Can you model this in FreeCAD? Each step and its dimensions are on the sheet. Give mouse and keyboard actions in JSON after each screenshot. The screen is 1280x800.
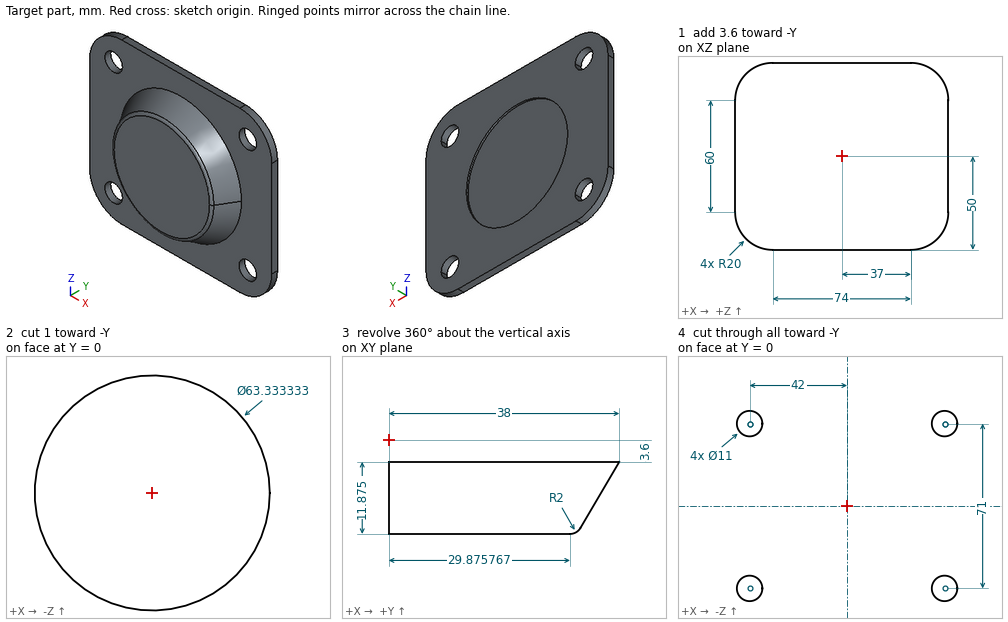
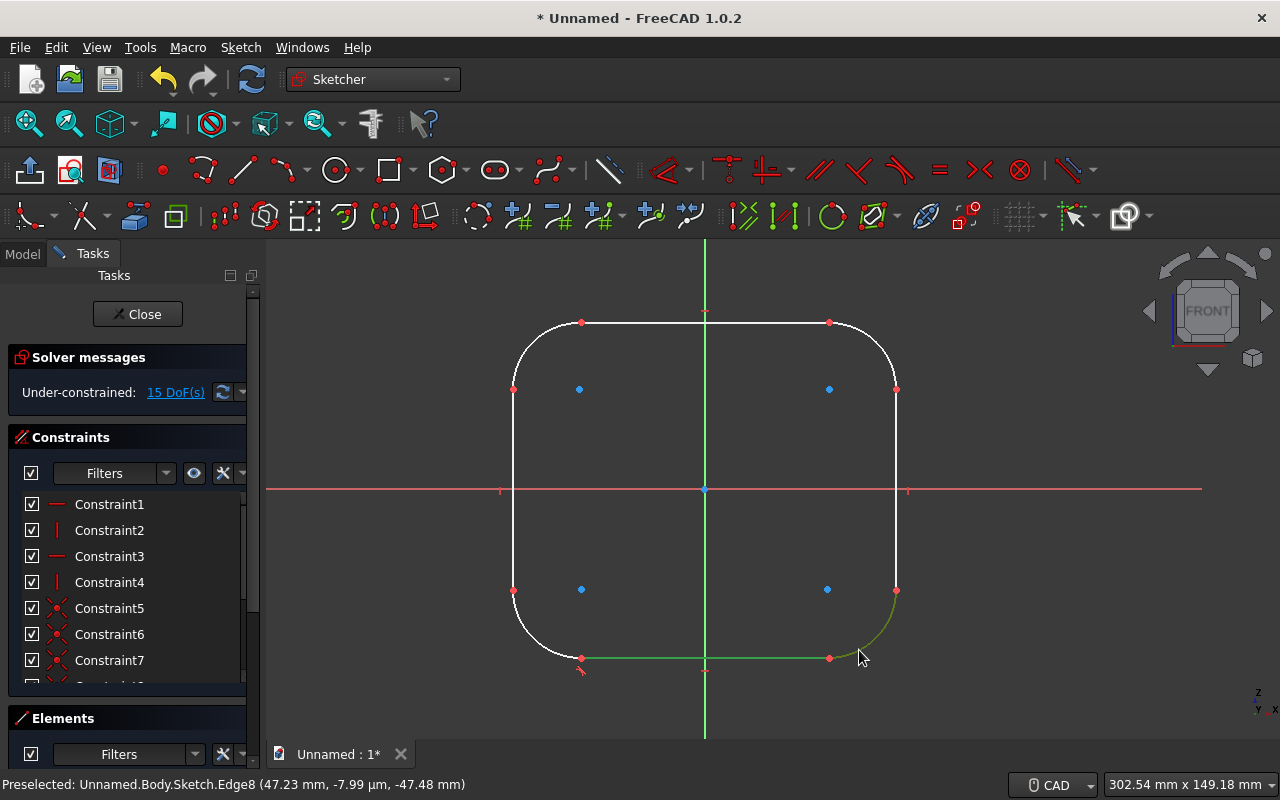
{"action": "left_click", "coordinate": [900, 170]}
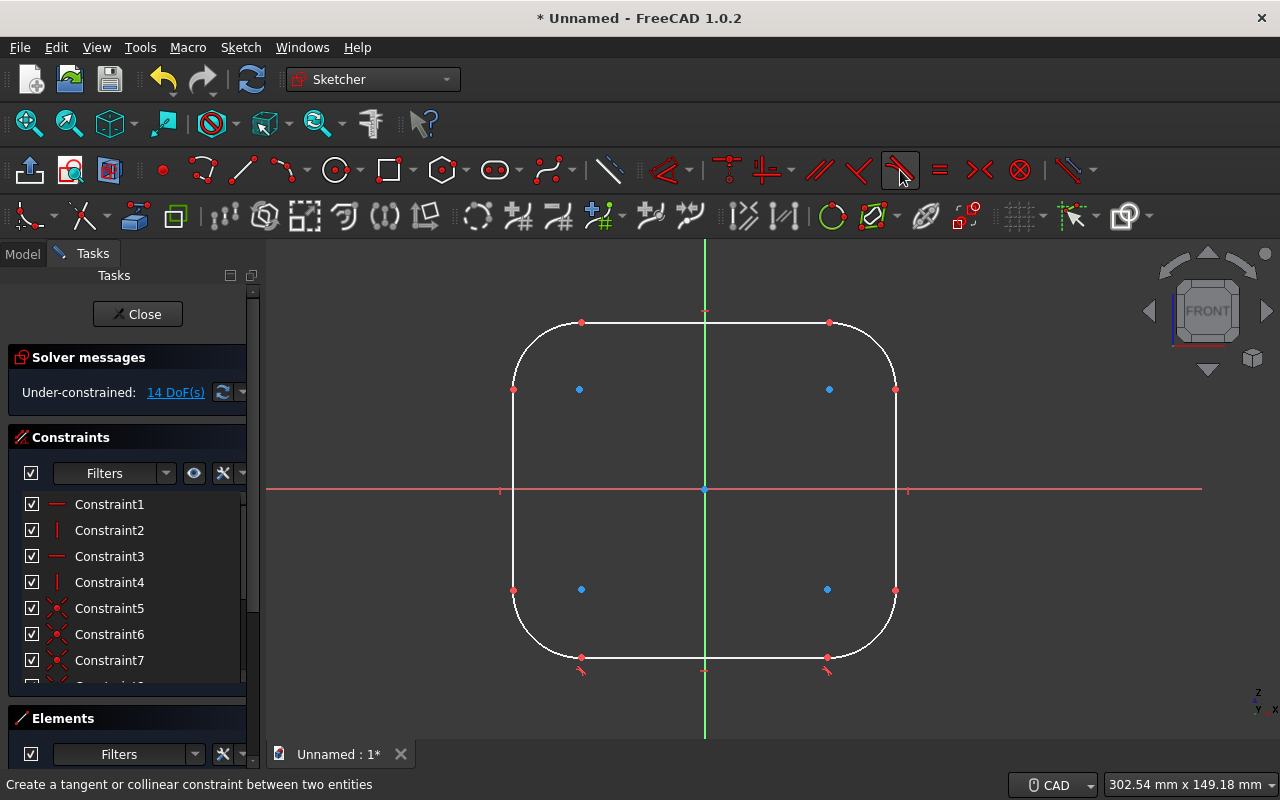
{"action": "left_click", "coordinate": [513, 531]}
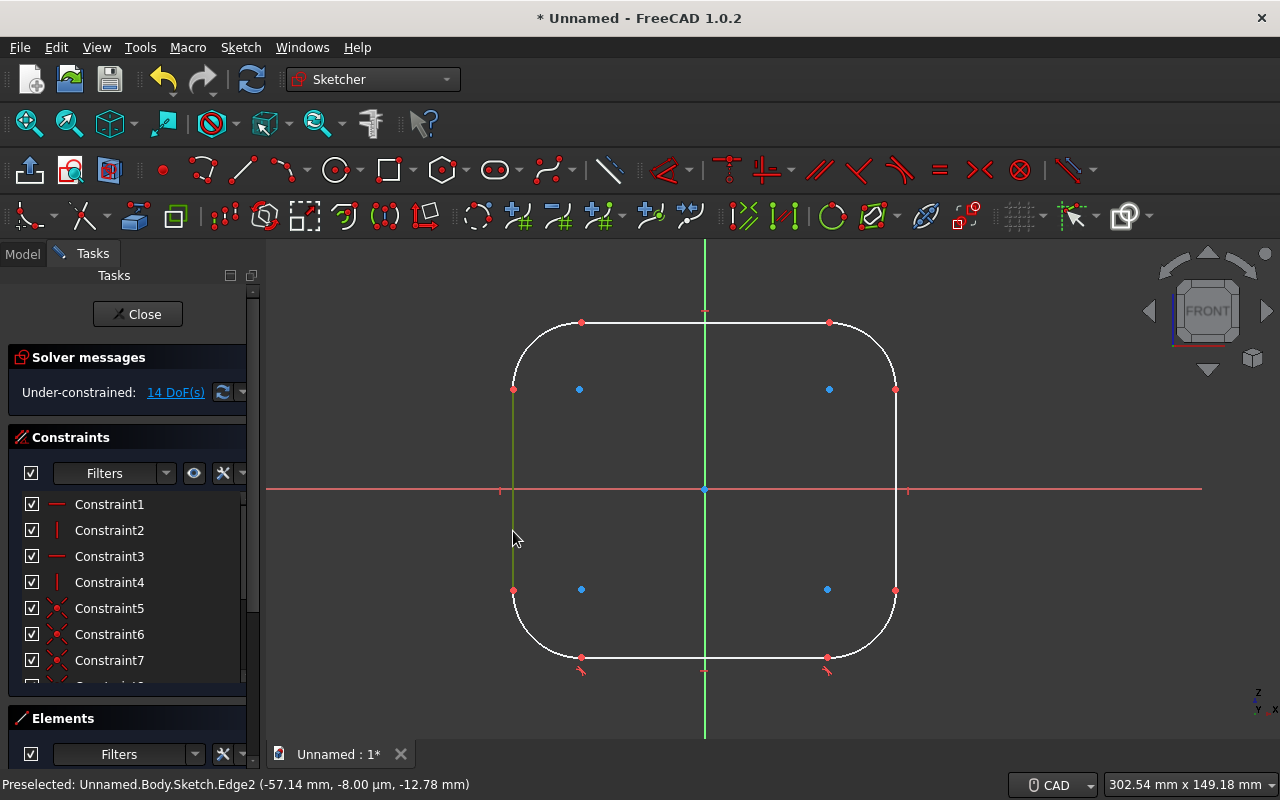
{"action": "left_click", "coordinate": [521, 622]}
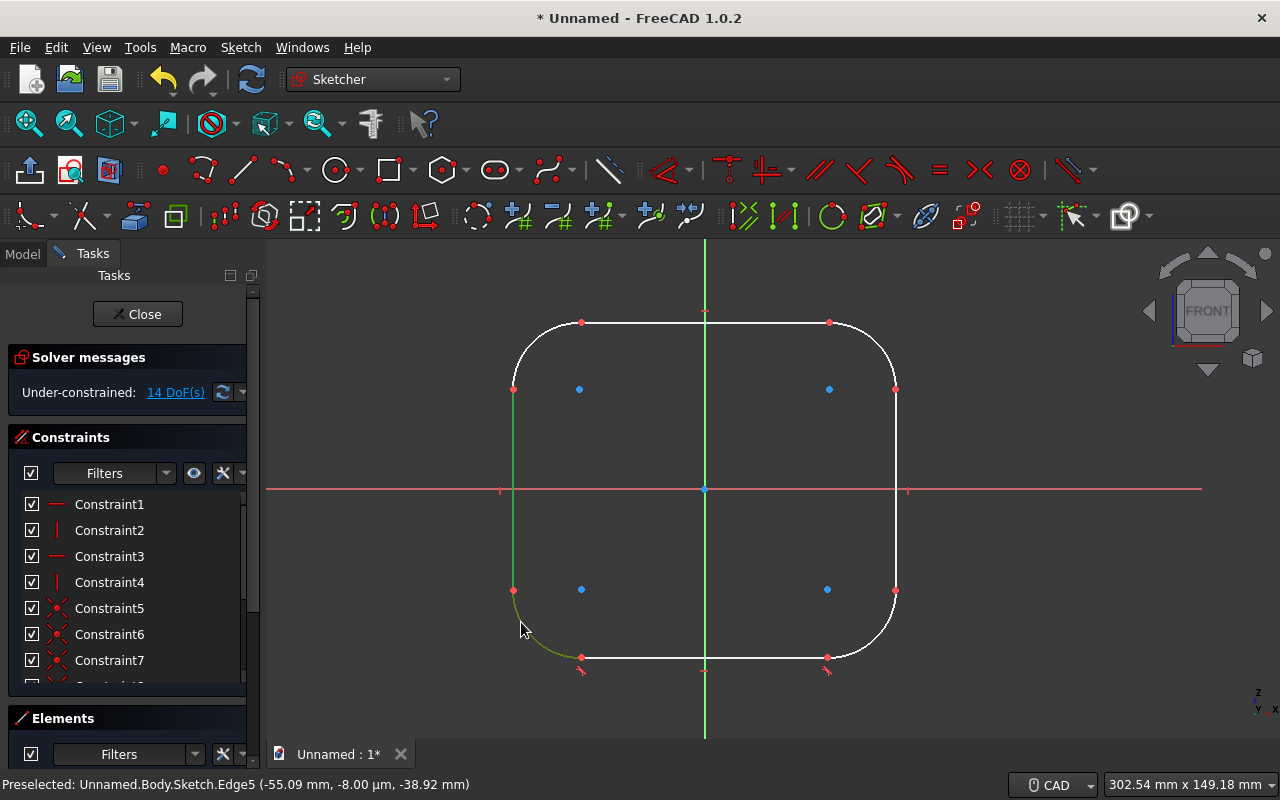
{"action": "left_click", "coordinate": [900, 170]}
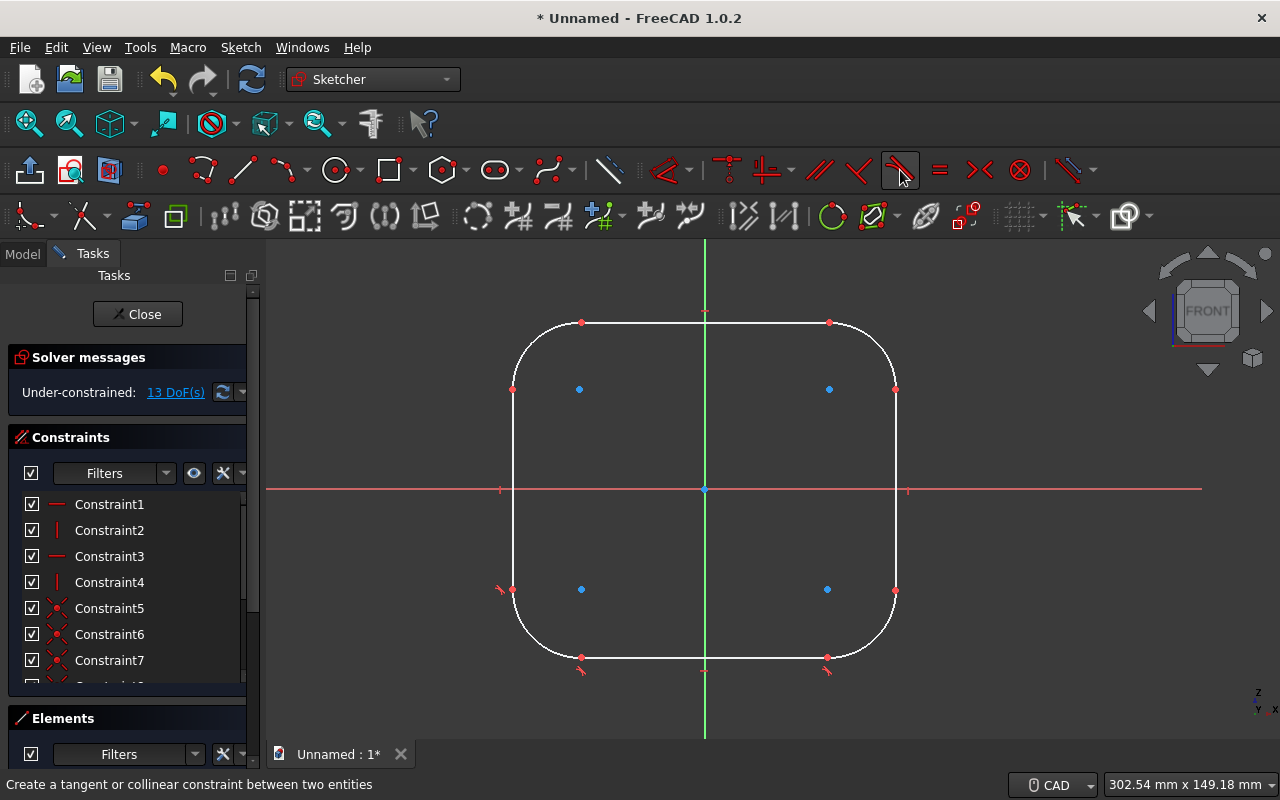
{"action": "left_click", "coordinate": [513, 530]}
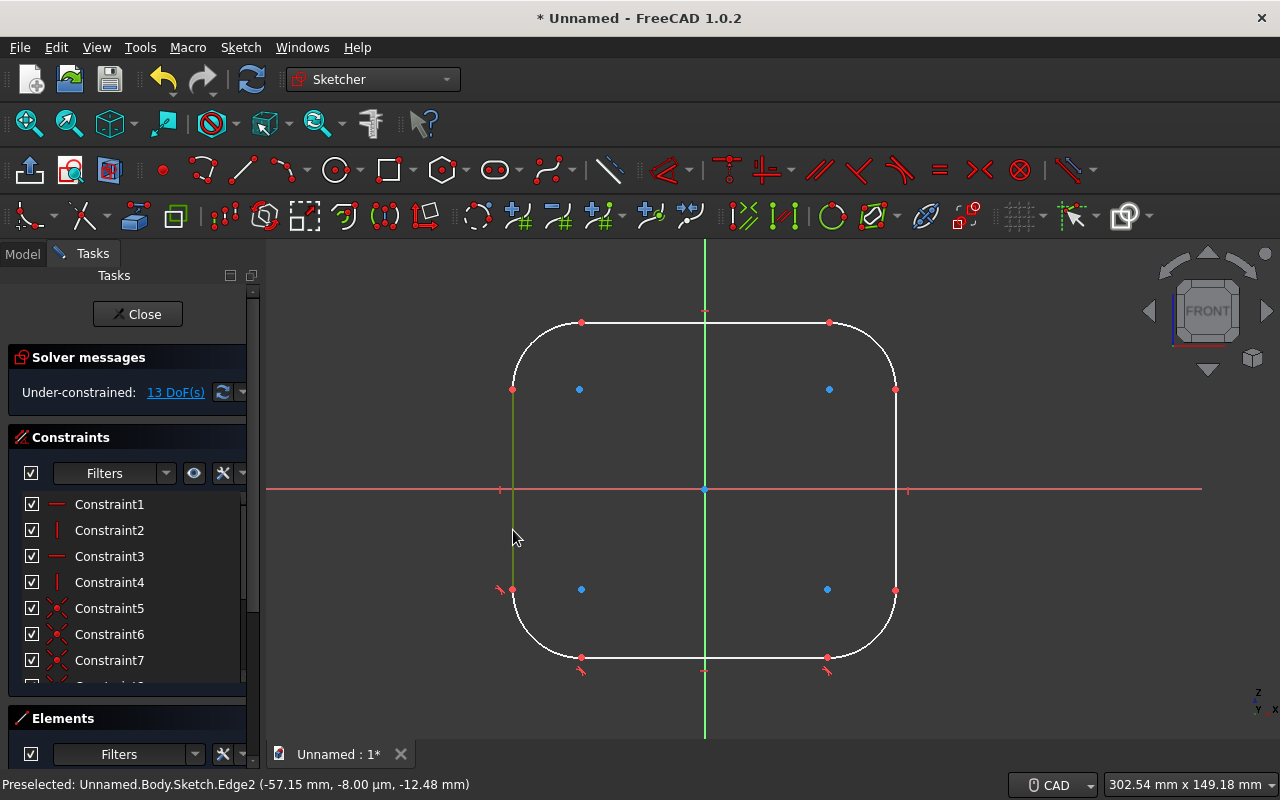
{"action": "left_click", "coordinate": [550, 330]}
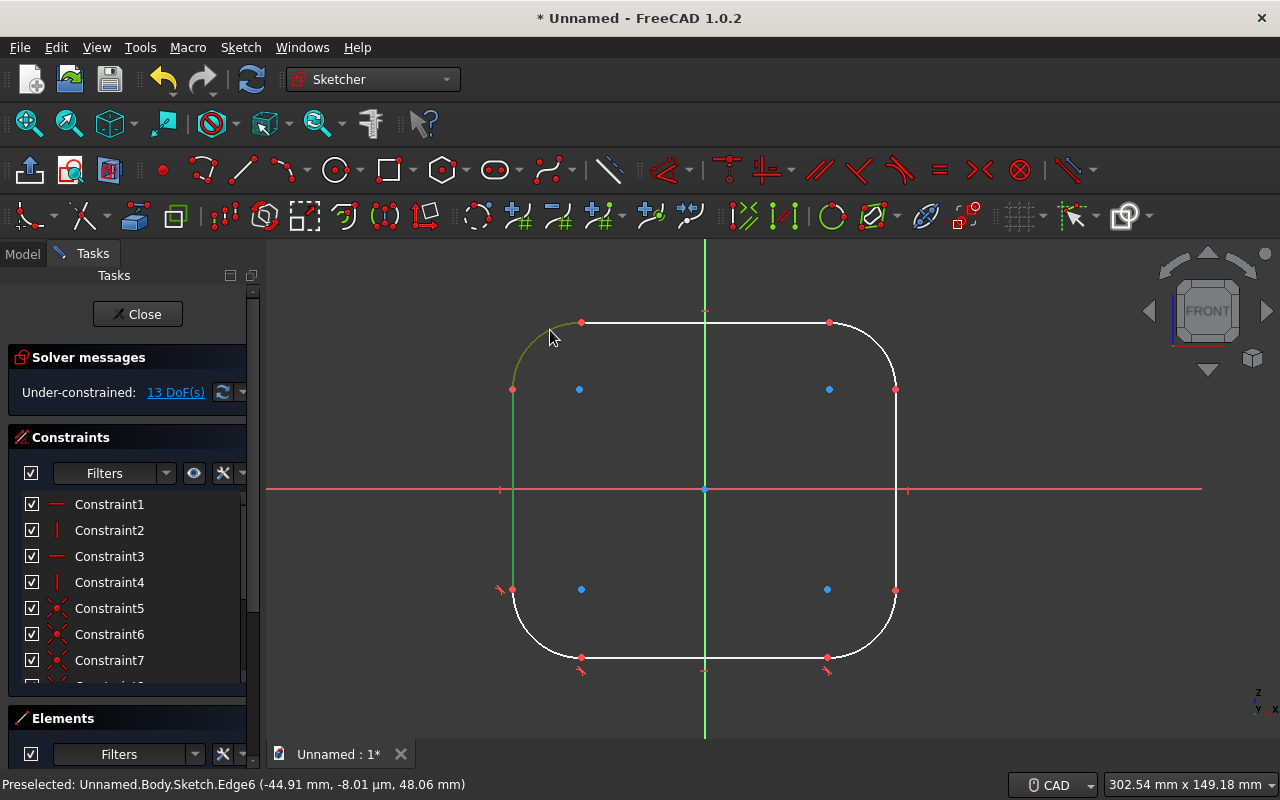
{"action": "left_click", "coordinate": [900, 170]}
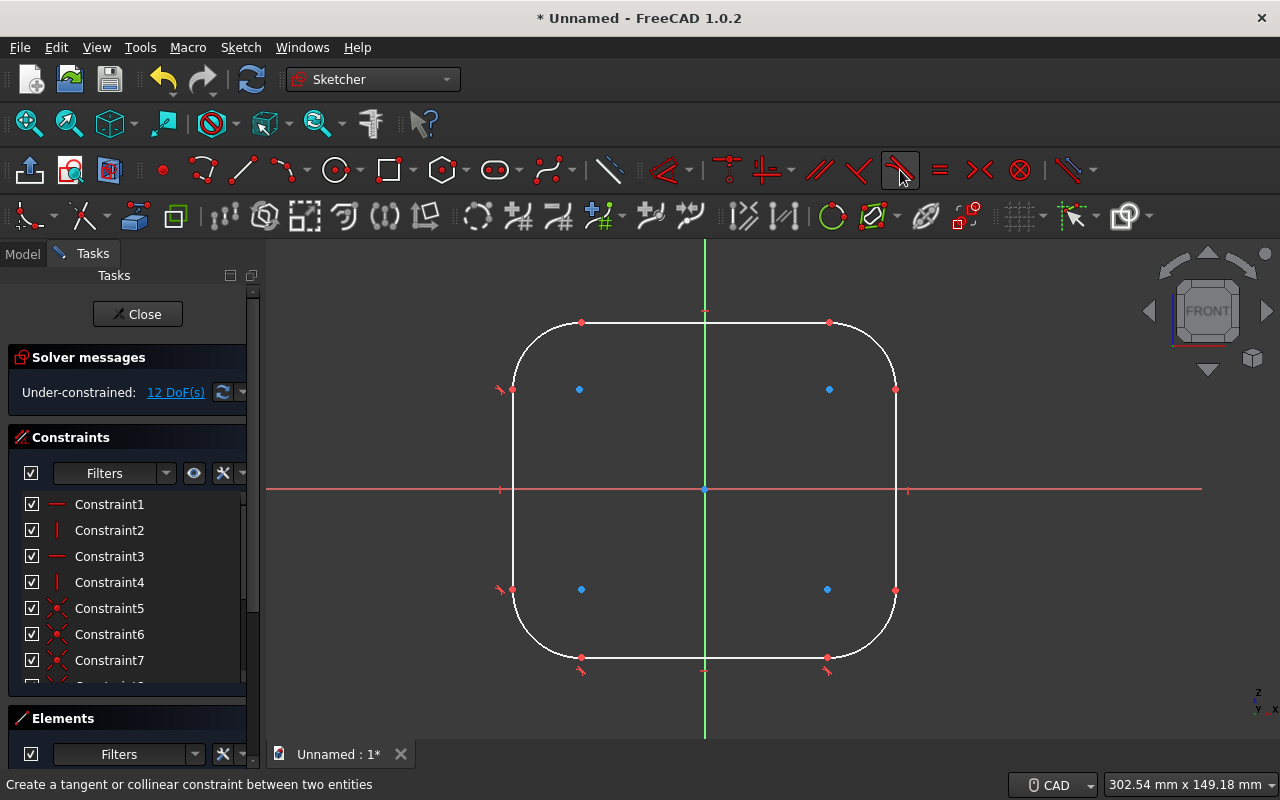
{"action": "left_click", "coordinate": [655, 323]}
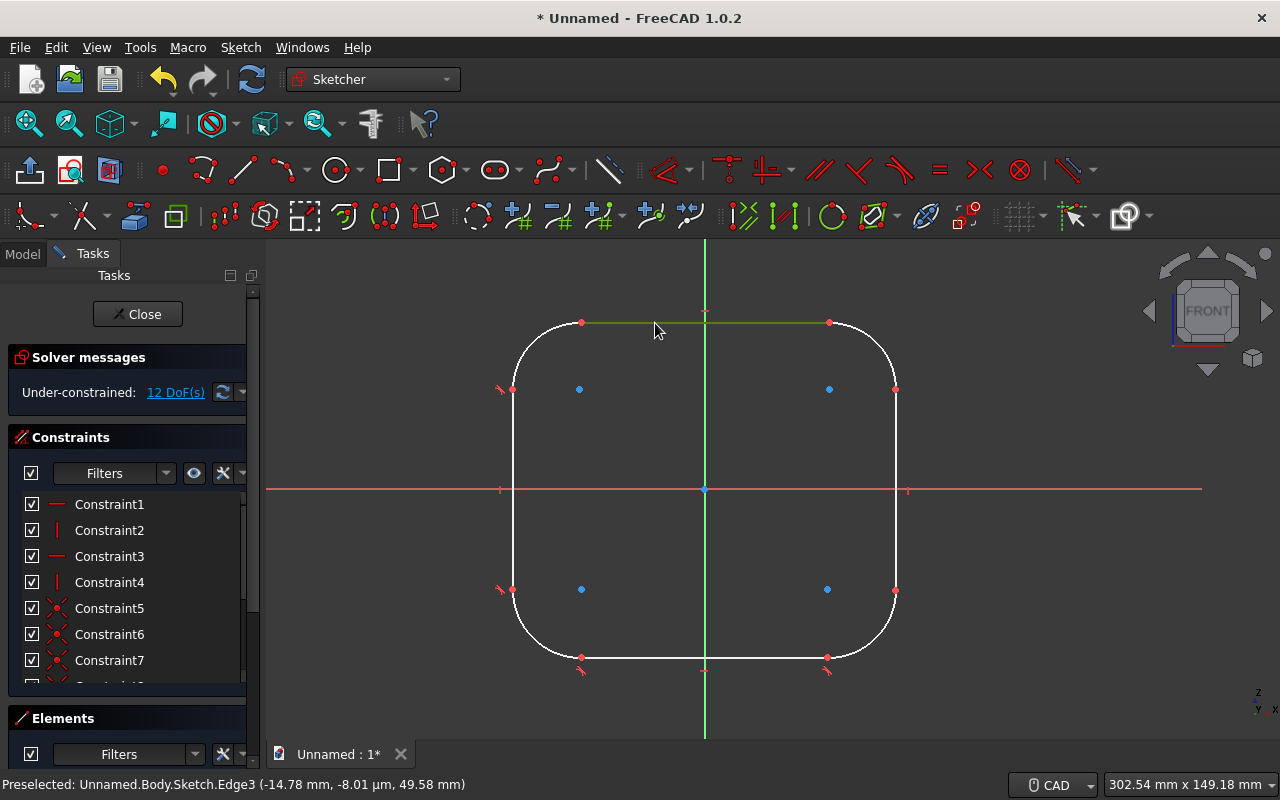
{"action": "left_click", "coordinate": [550, 330]}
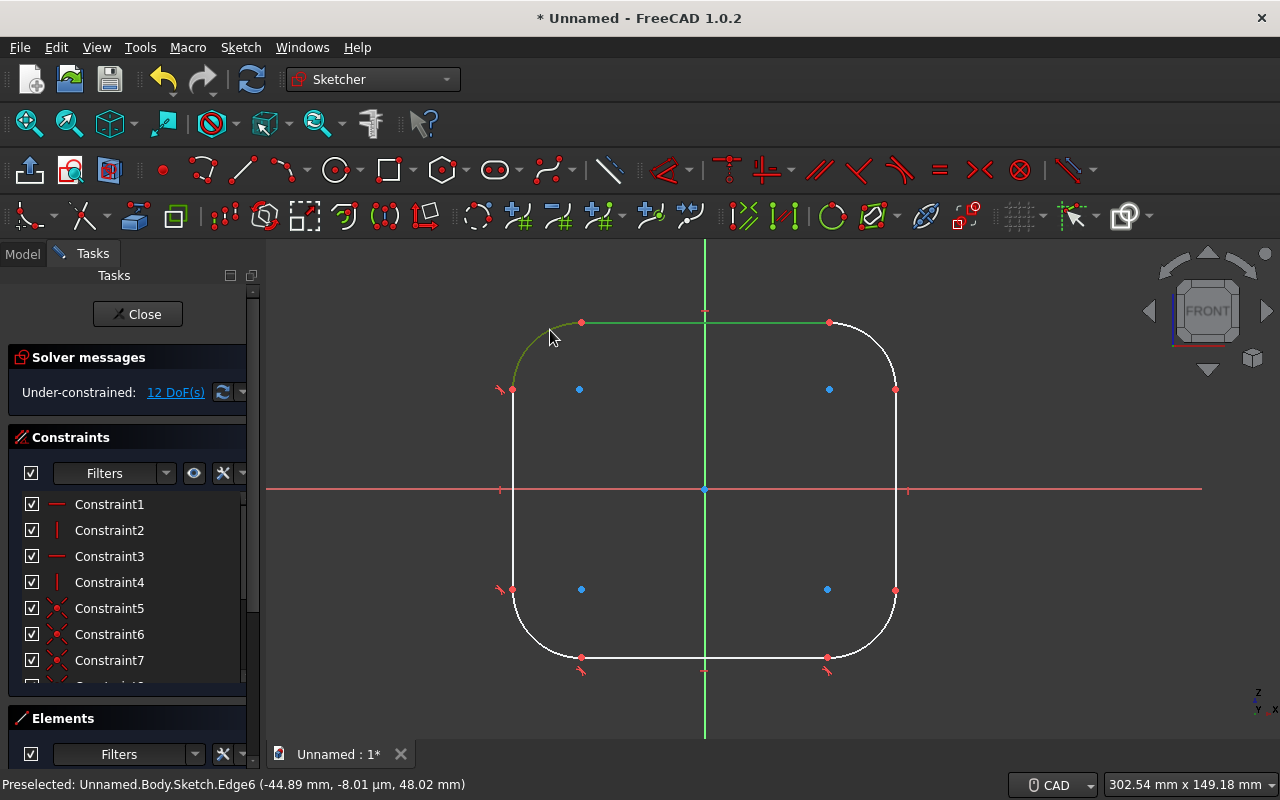
{"action": "left_click", "coordinate": [900, 170]}